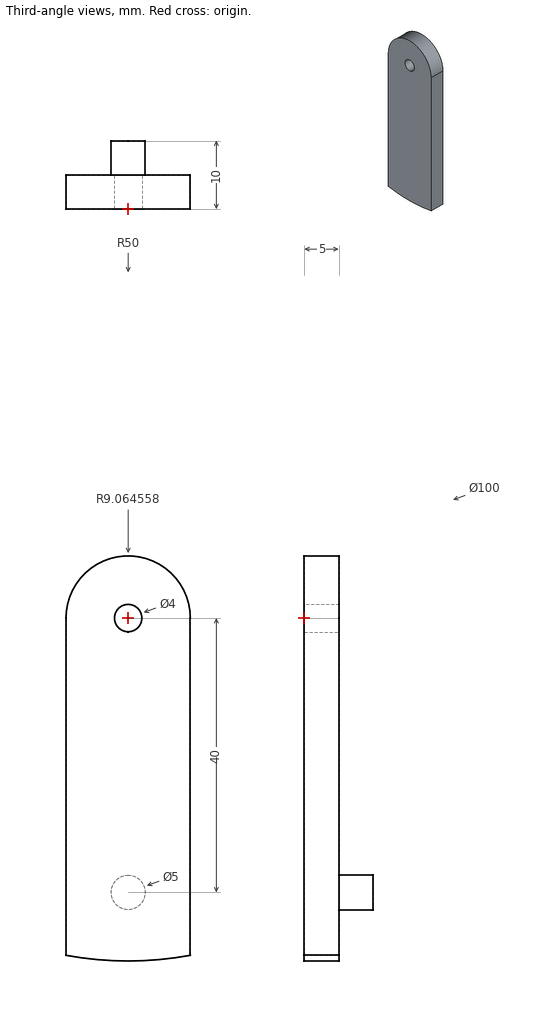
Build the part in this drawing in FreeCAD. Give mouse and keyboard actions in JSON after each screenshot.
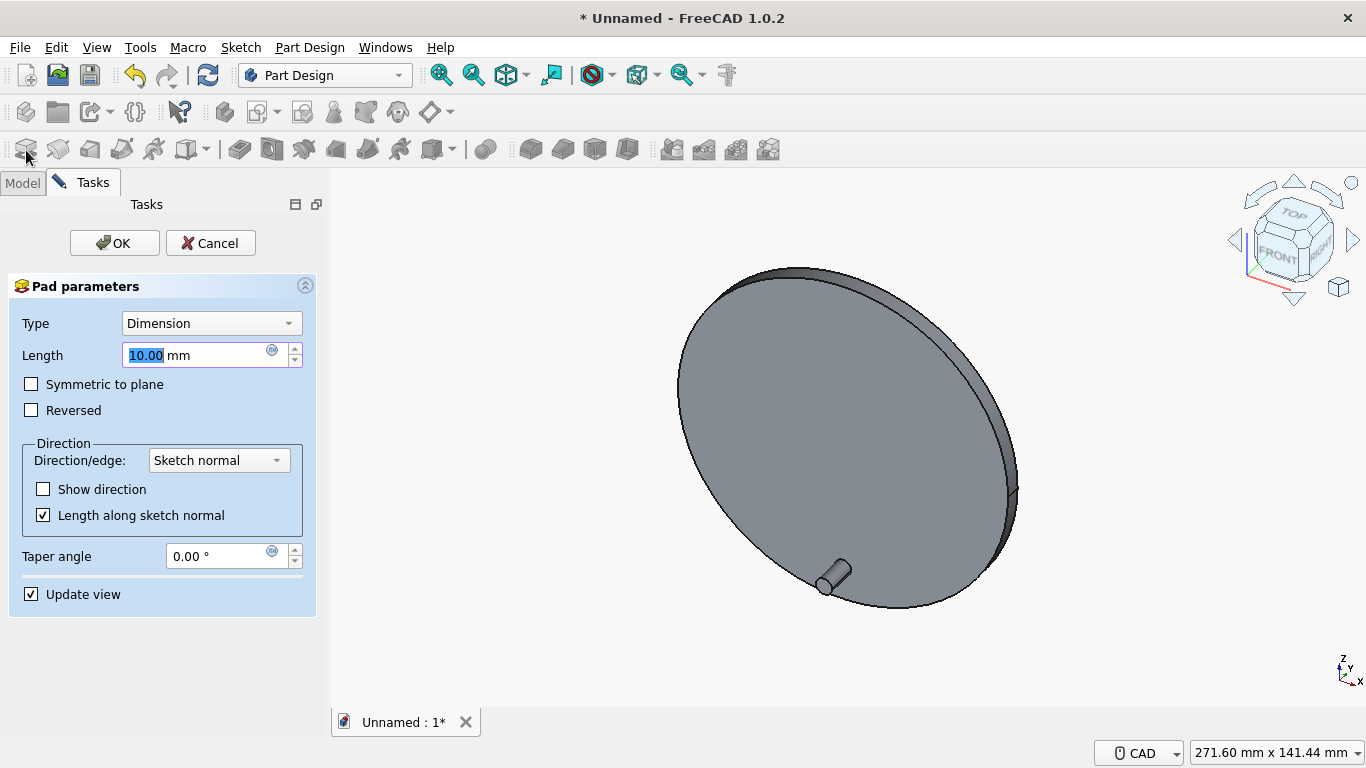
{"action": "type", "text": "10"}
{"action": "key", "text": "Tab"}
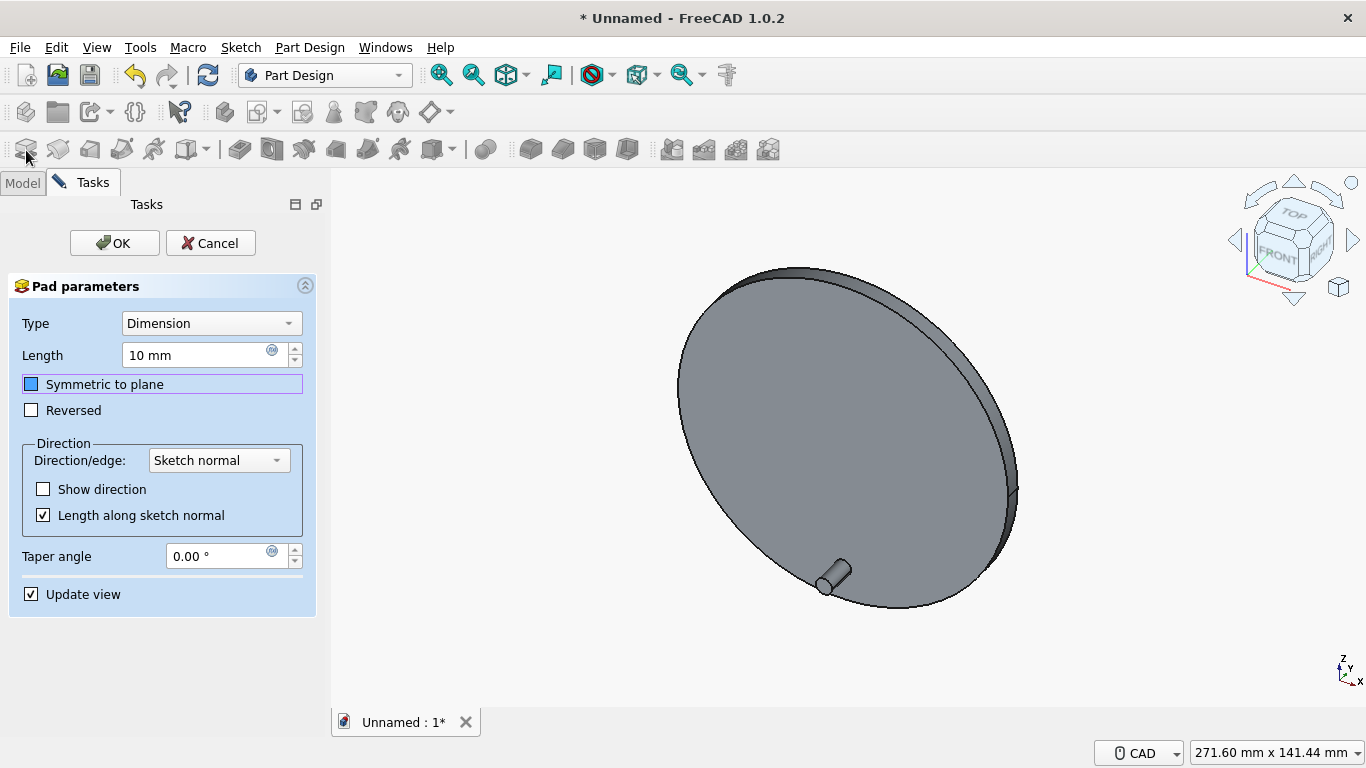
{"action": "left_click", "coordinate": [30, 410]}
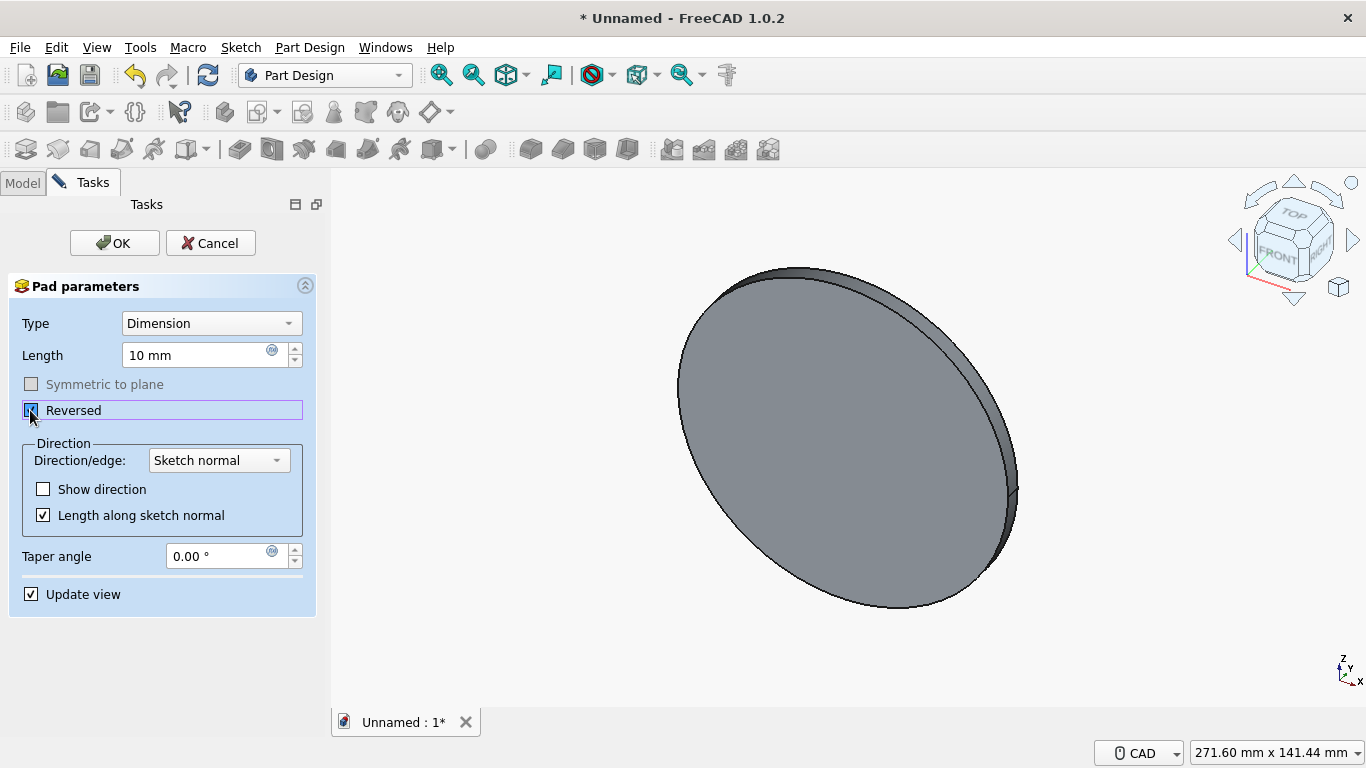
{"action": "left_click", "coordinate": [115, 243]}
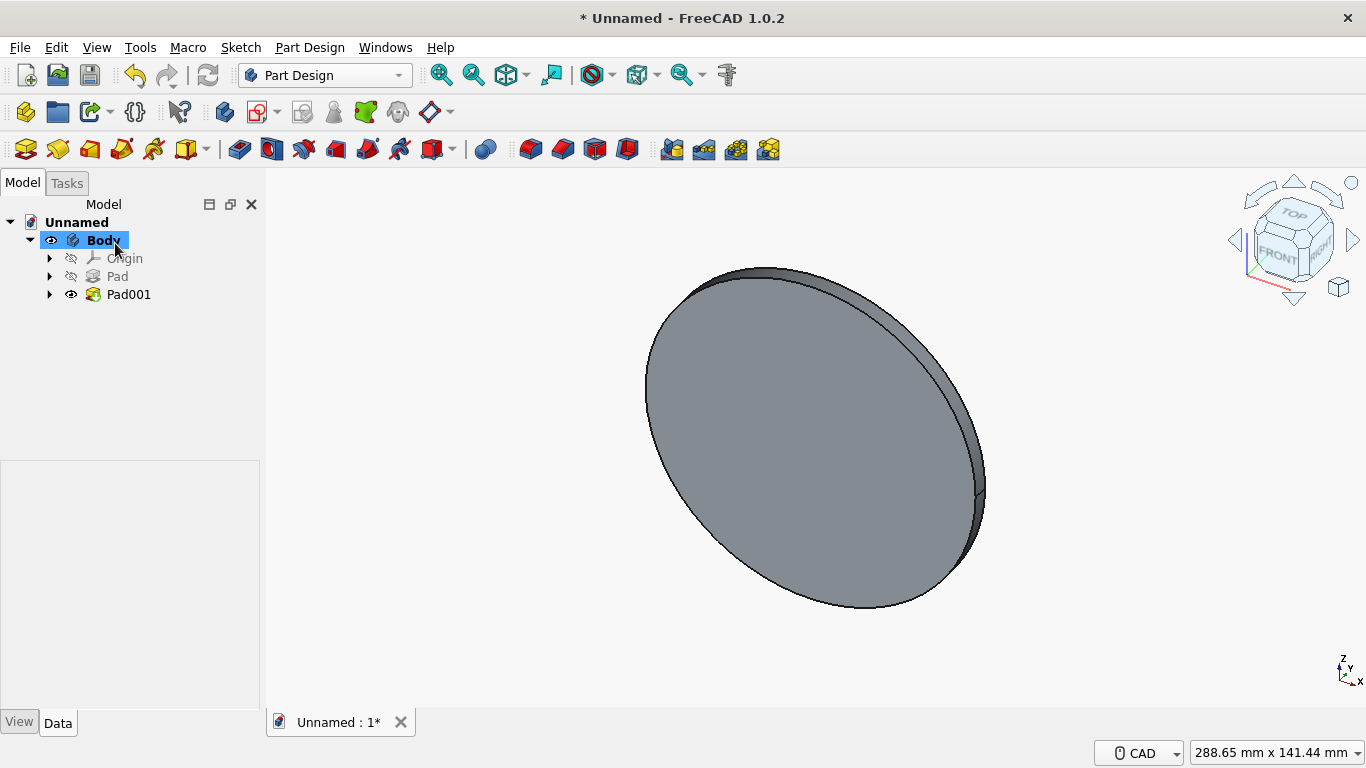
{"action": "left_click", "coordinate": [50, 258]}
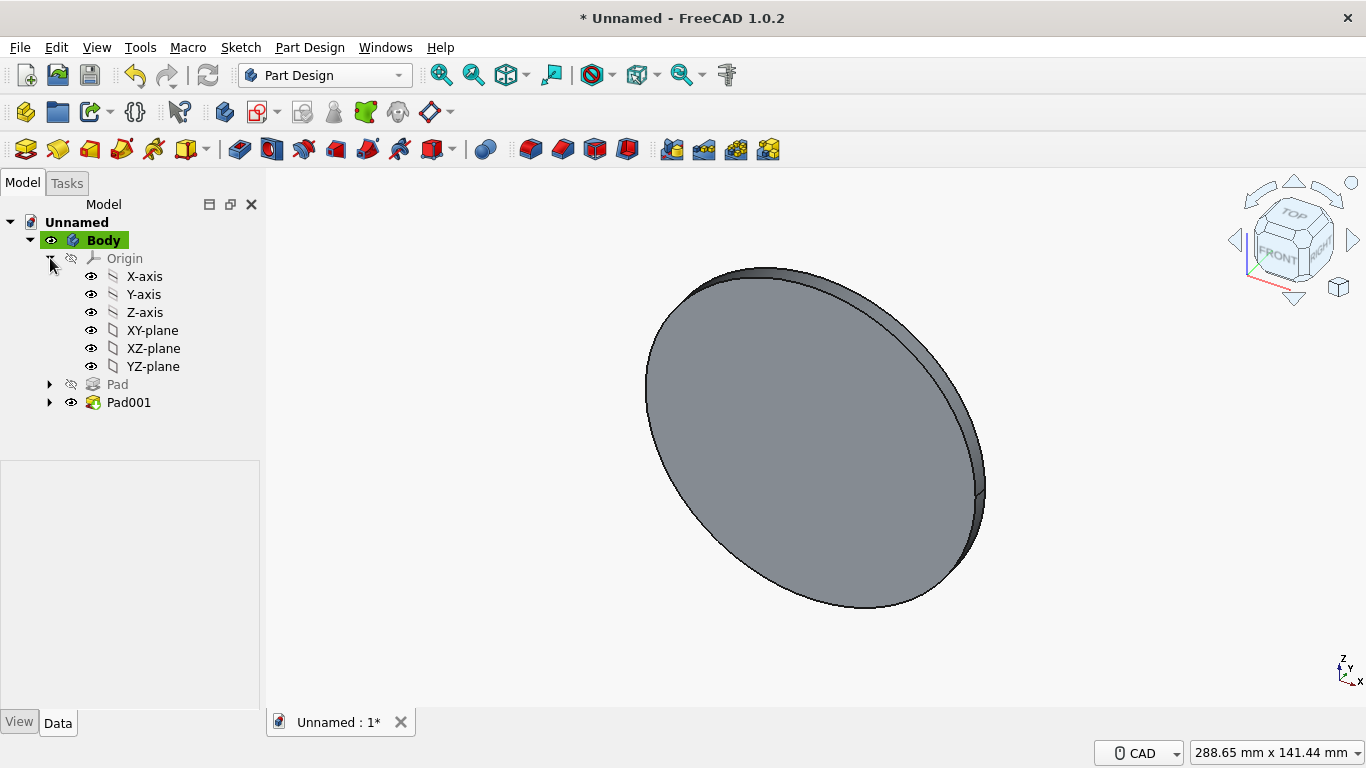
{"action": "left_click", "coordinate": [136, 348]}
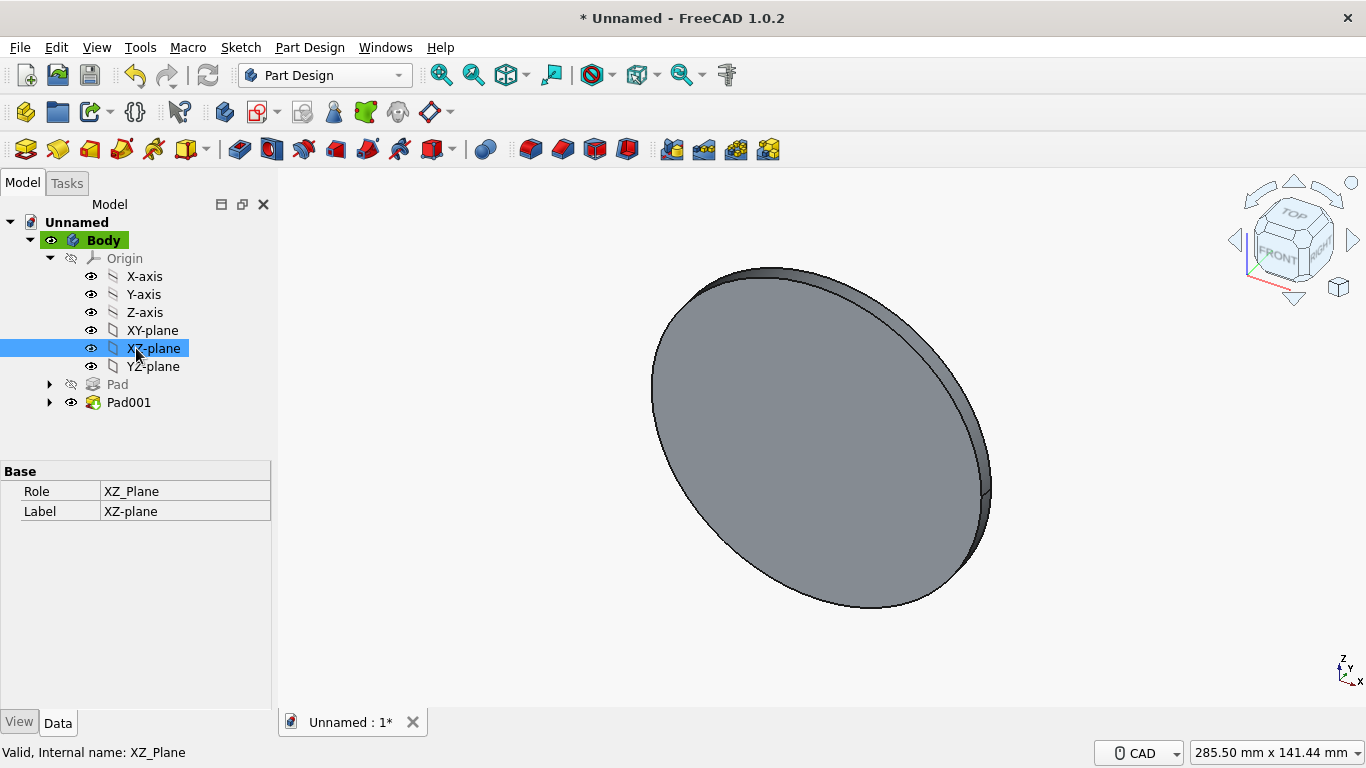
{"action": "left_click", "coordinate": [430, 112]}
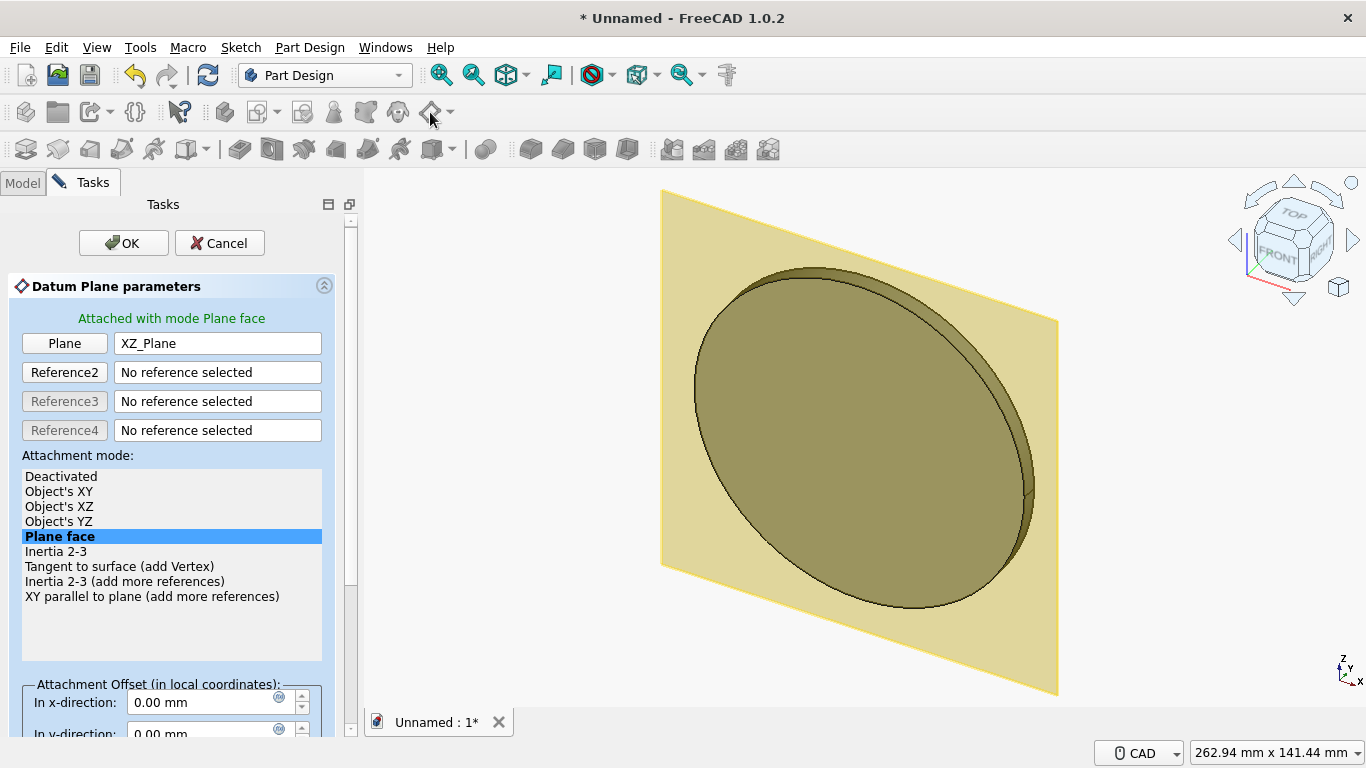
{"action": "scroll", "coordinate": [351, 475], "scroll_direction": "down", "scroll_amount": 2}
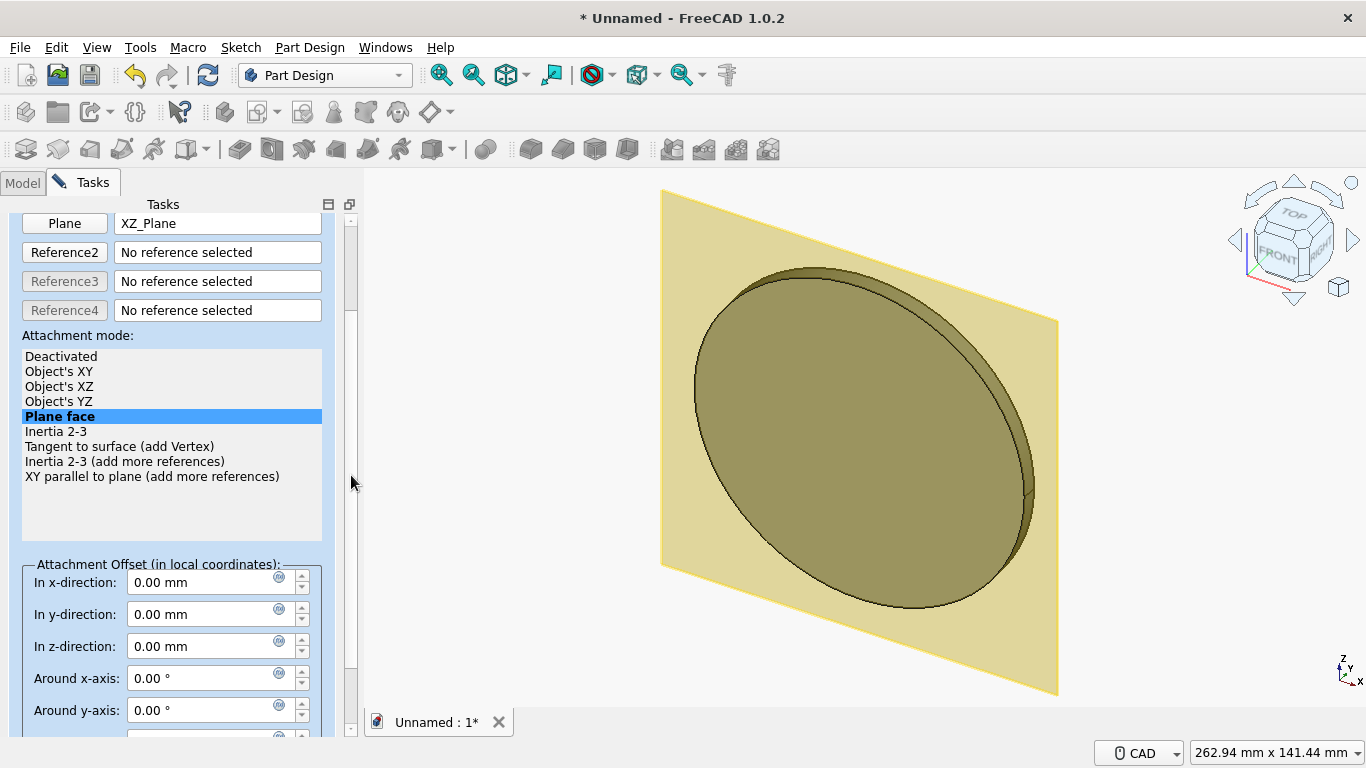
{"action": "triple_click", "coordinate": [210, 646]}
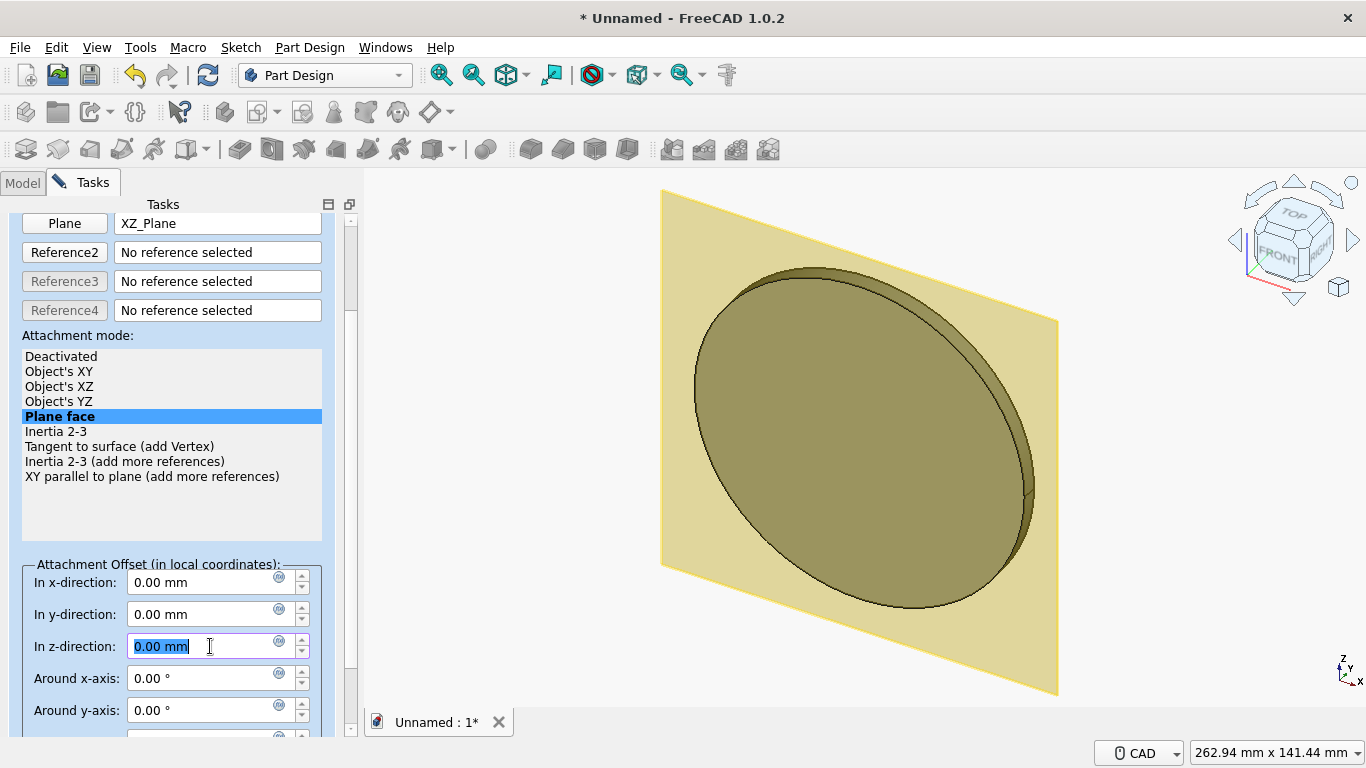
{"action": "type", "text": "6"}
{"action": "key", "text": "Tab"}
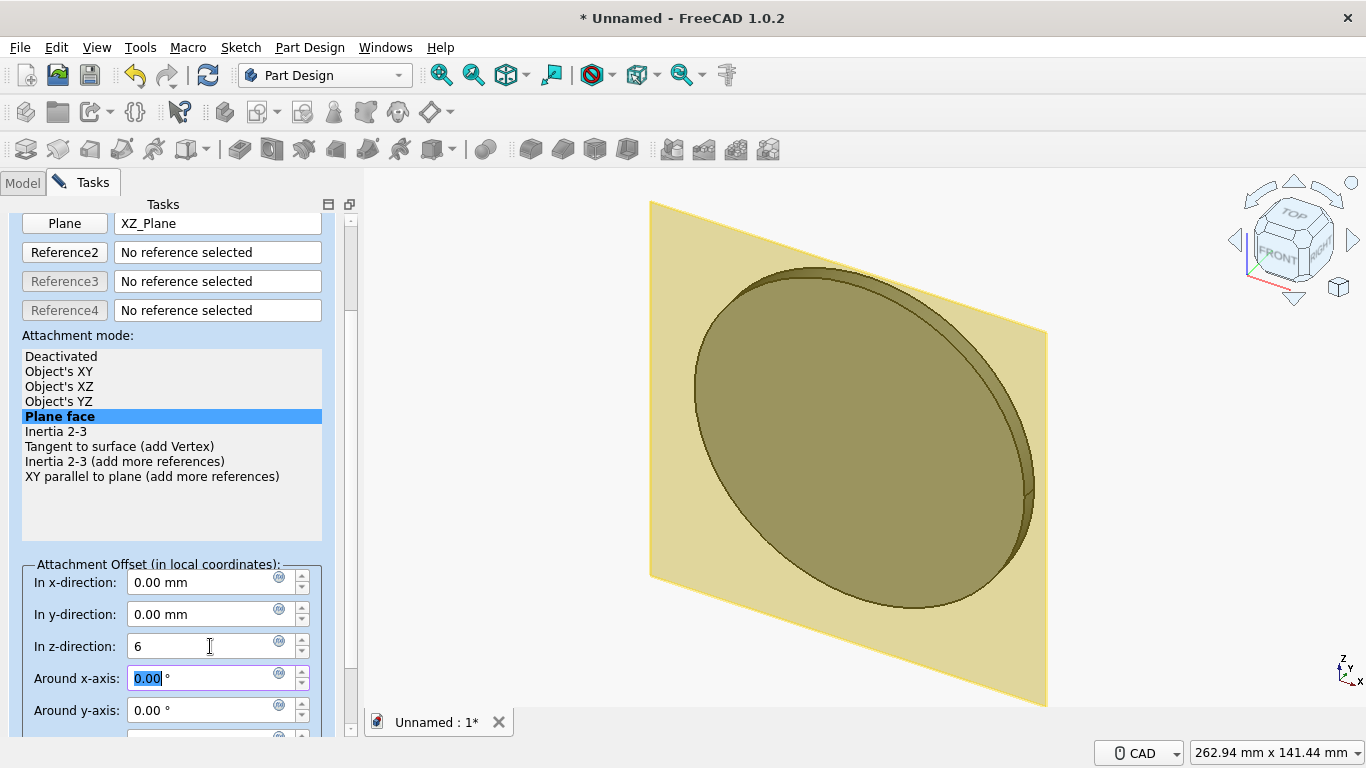
{"action": "scroll", "coordinate": [351, 475], "scroll_direction": "up", "scroll_amount": 3}